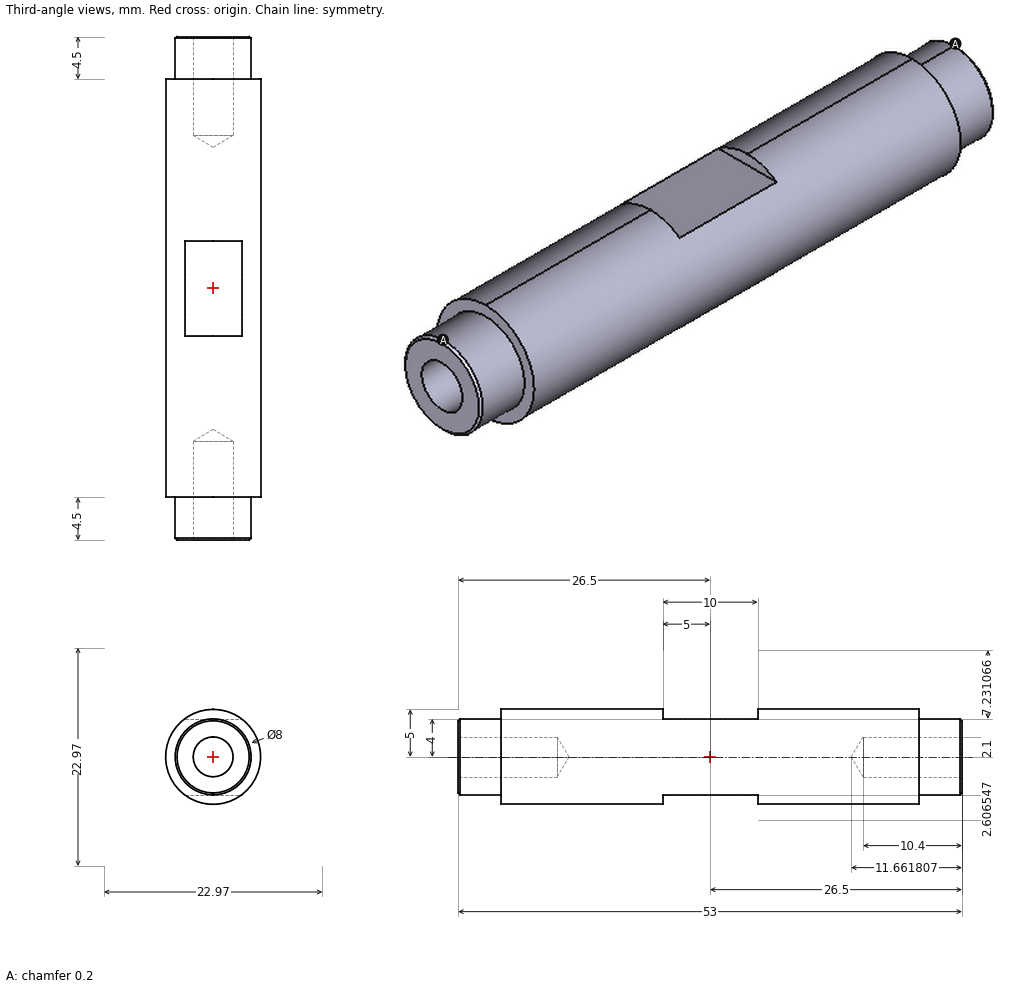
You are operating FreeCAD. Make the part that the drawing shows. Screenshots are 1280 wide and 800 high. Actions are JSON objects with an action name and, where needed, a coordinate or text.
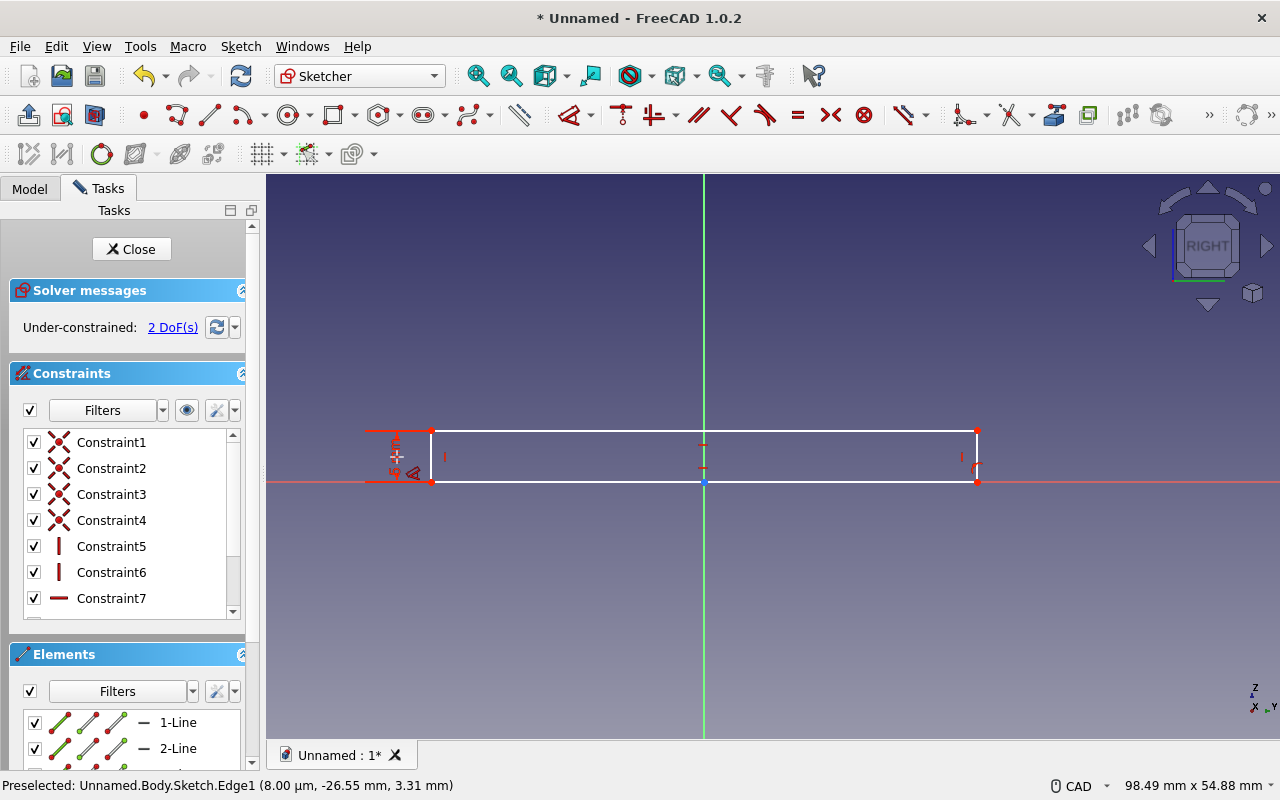
{"action": "left_click", "coordinate": [595, 482]}
{"action": "left_click", "coordinate": [578, 516]}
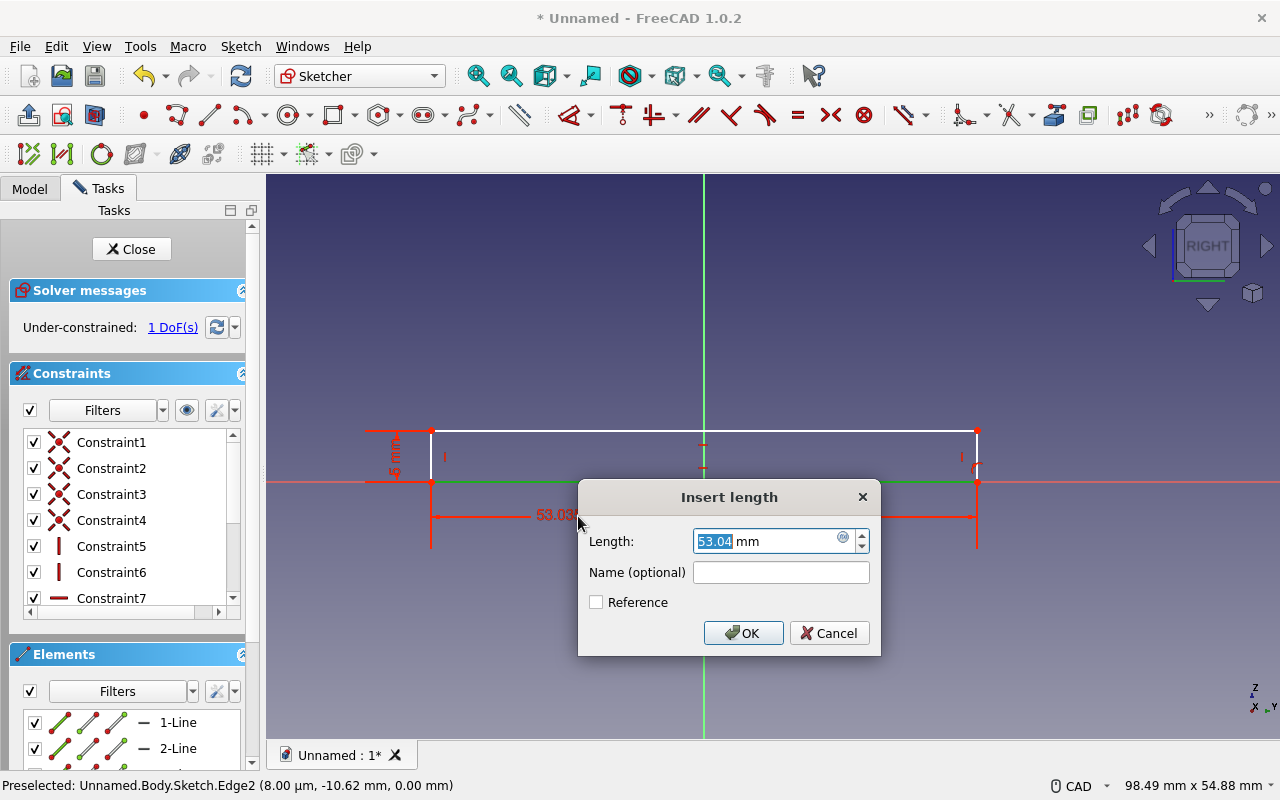
{"action": "type", "text": "53"}
{"action": "key", "text": "Return"}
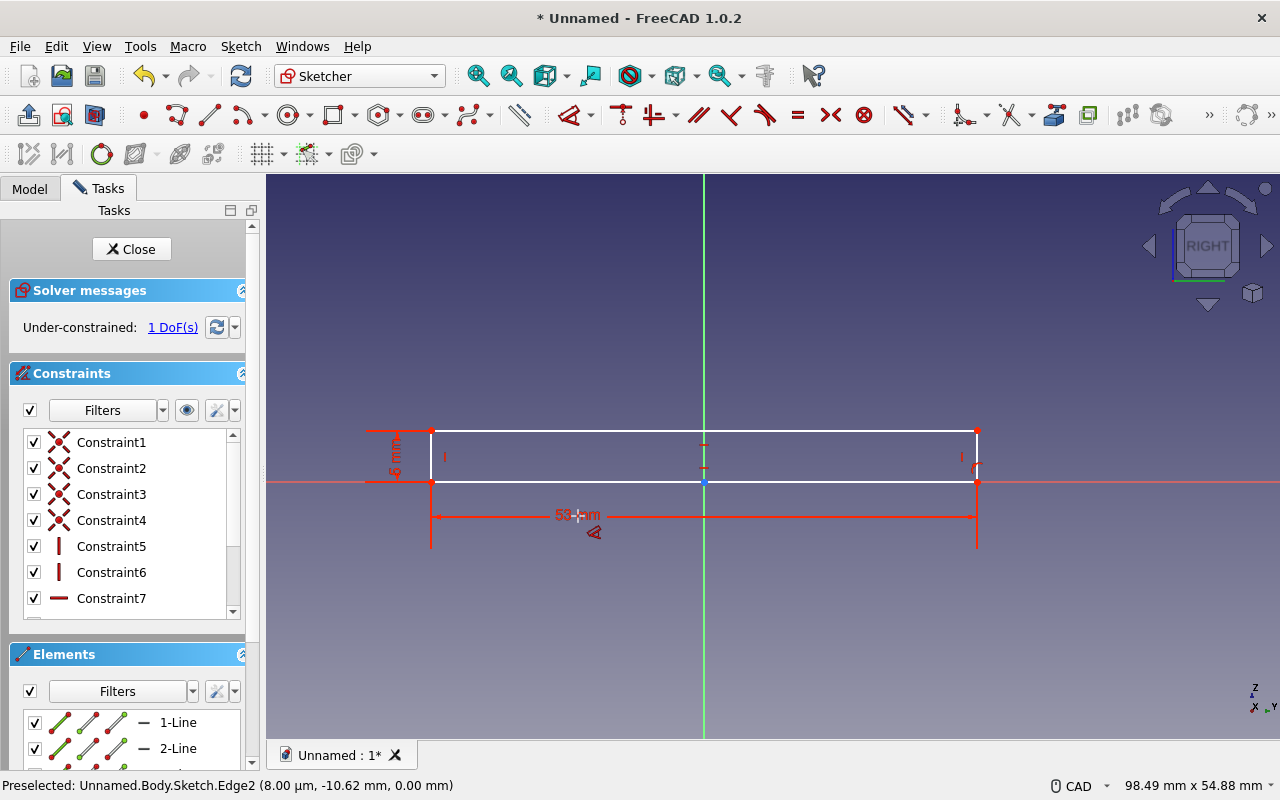
{"action": "left_click", "coordinate": [431, 431]}
{"action": "left_click", "coordinate": [568, 397]}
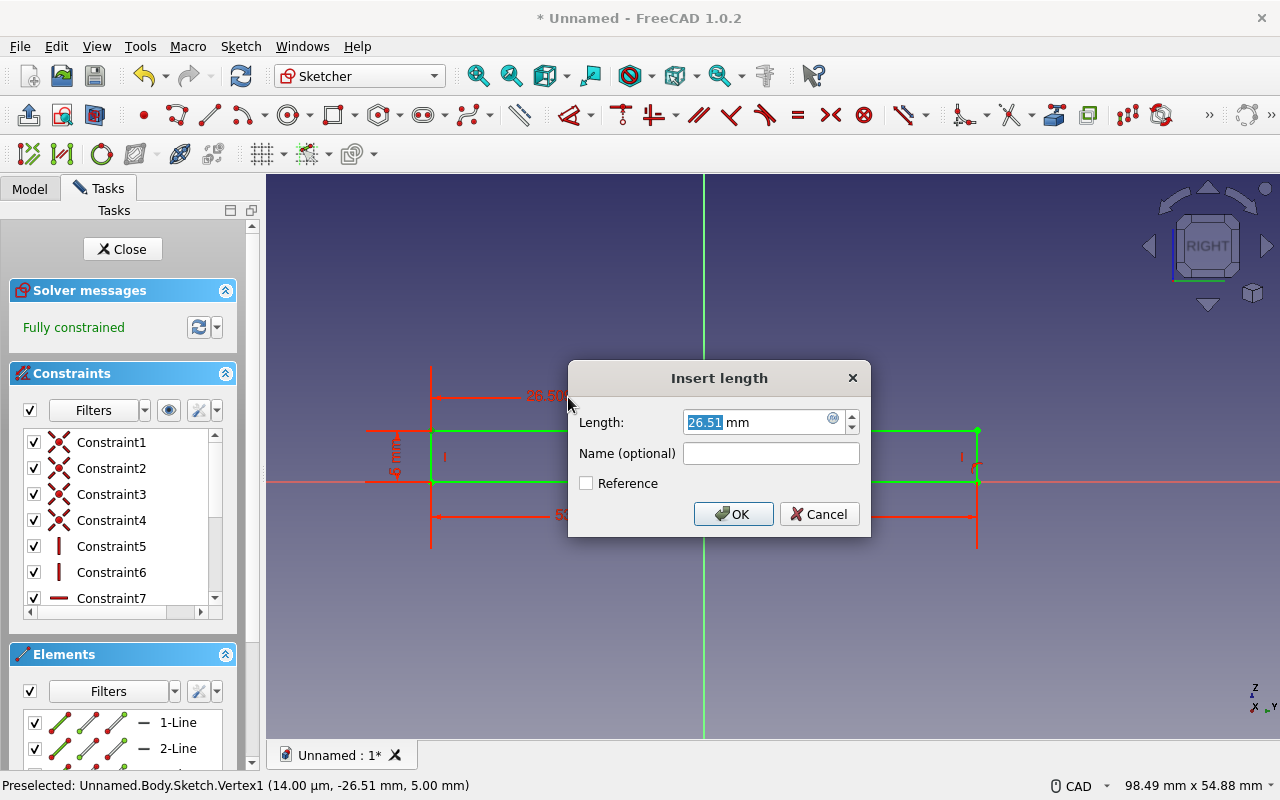
{"action": "type", "text": "26.5"}
{"action": "key", "text": "Return"}
{"action": "key", "text": "Escape"}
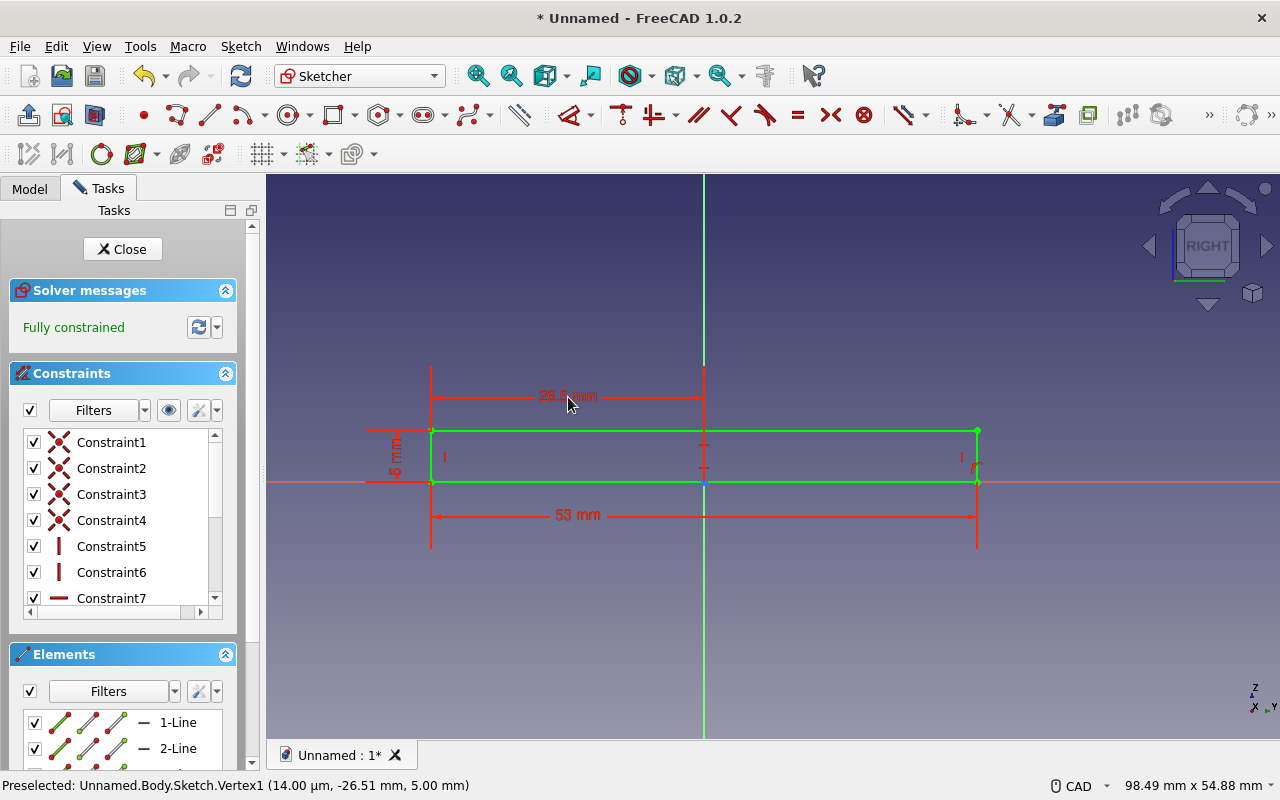
{"action": "left_click", "coordinate": [123, 249]}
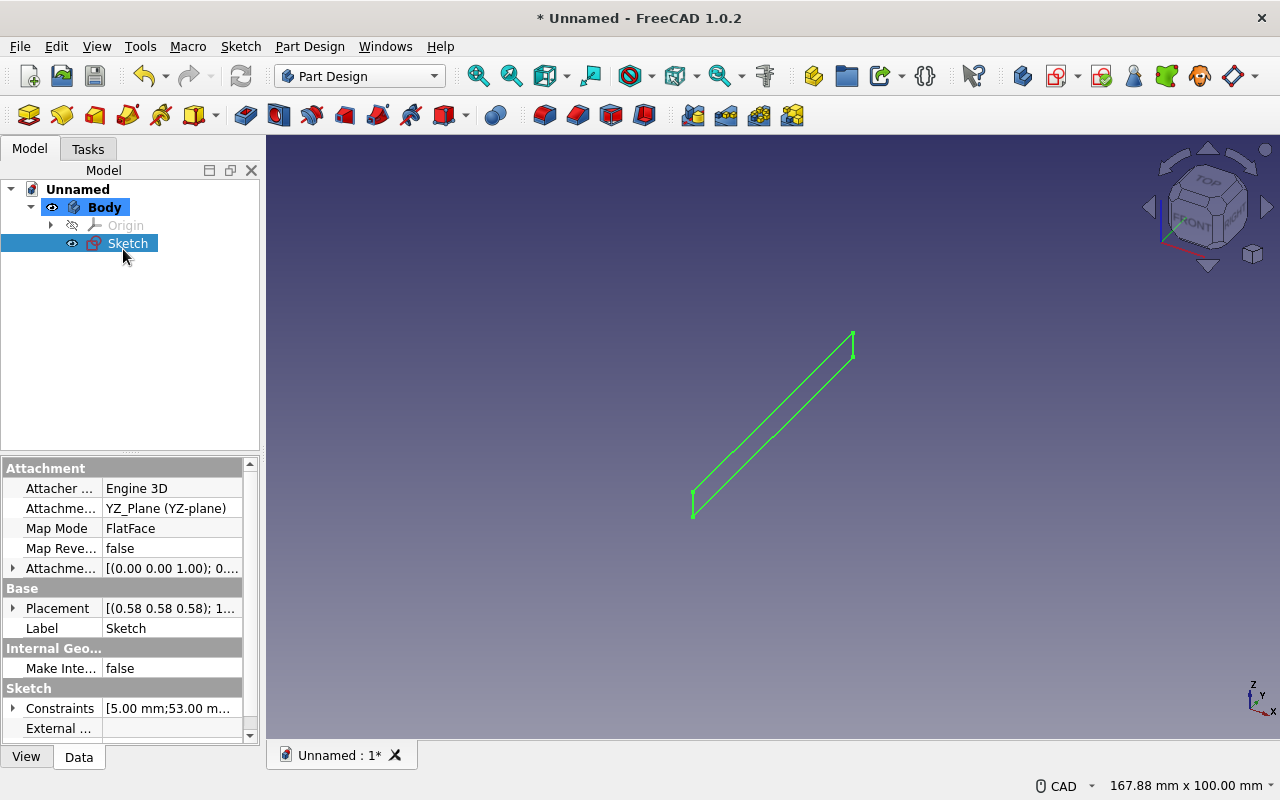
{"action": "left_click", "coordinate": [62, 116]}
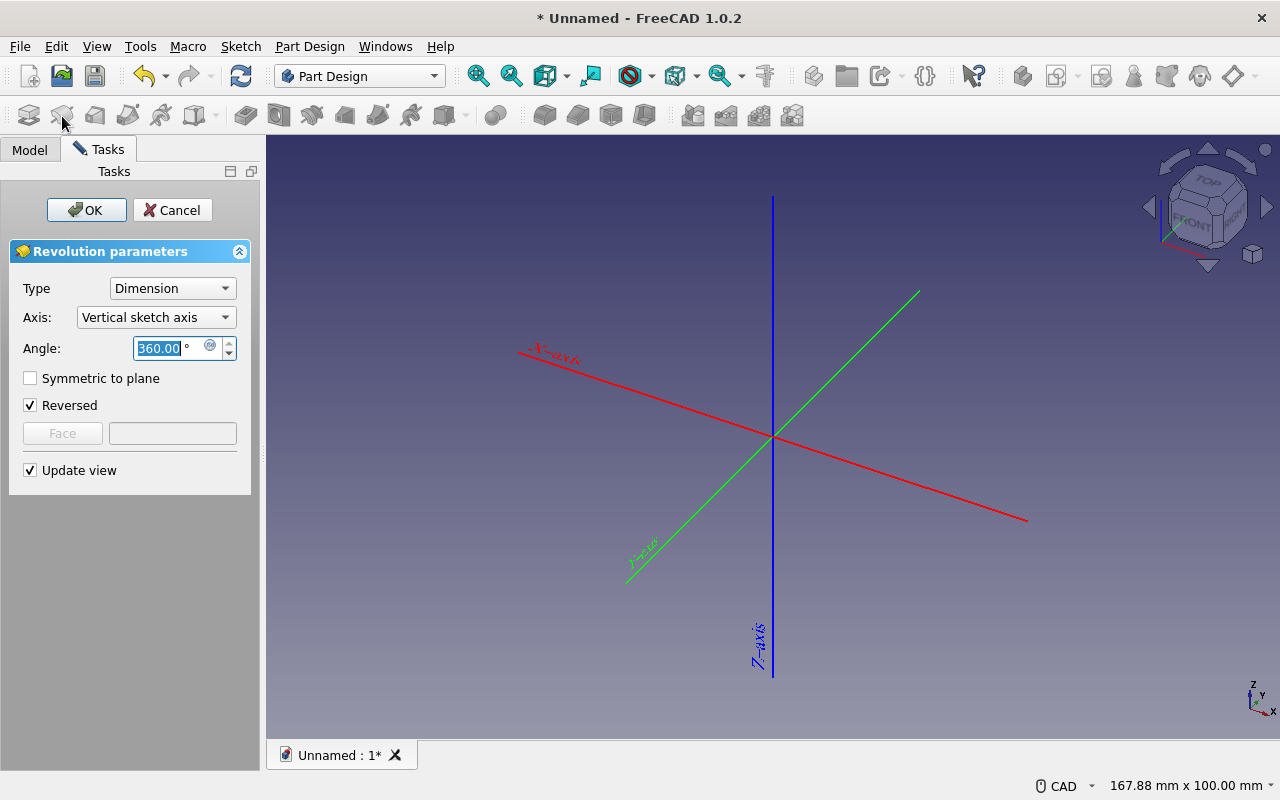
{"action": "left_click", "coordinate": [157, 318]}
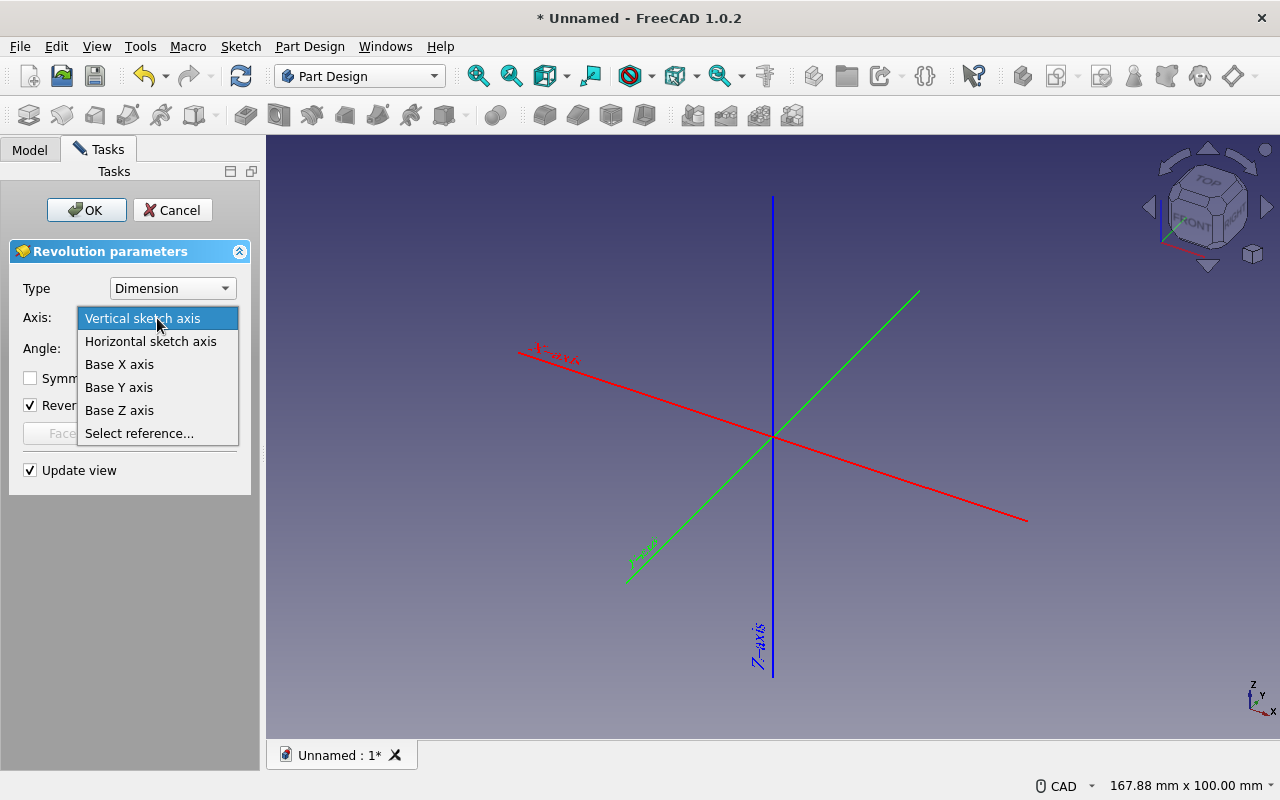
{"action": "left_click", "coordinate": [156, 342]}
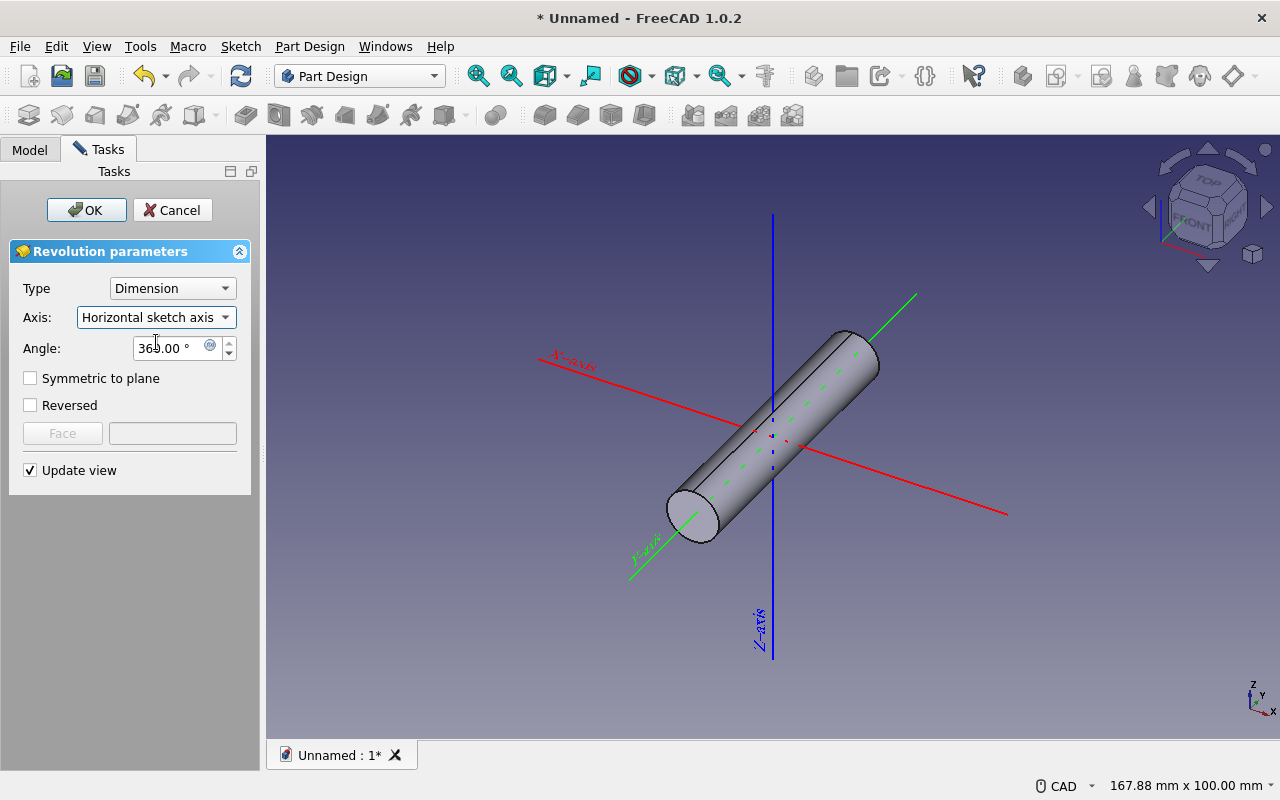
{"action": "left_click", "coordinate": [87, 210]}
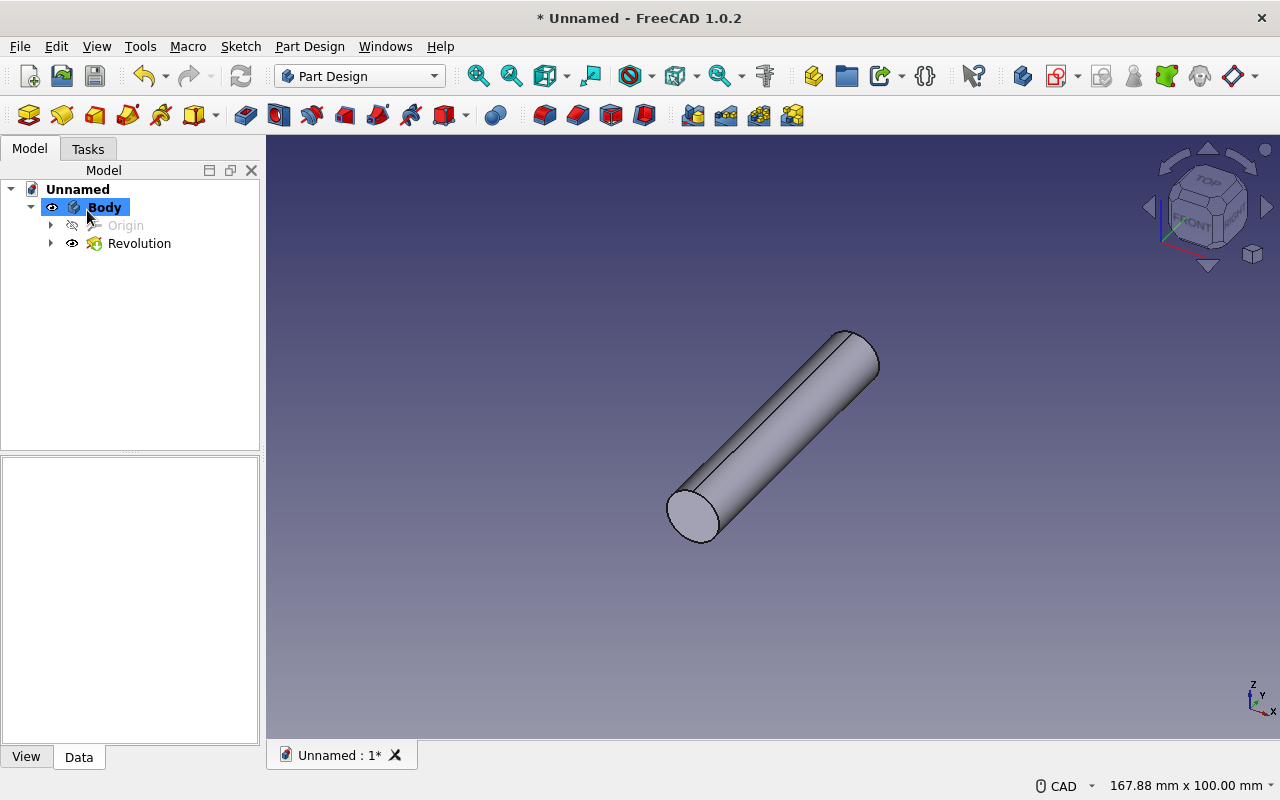
{"action": "left_click", "coordinate": [479, 76]}